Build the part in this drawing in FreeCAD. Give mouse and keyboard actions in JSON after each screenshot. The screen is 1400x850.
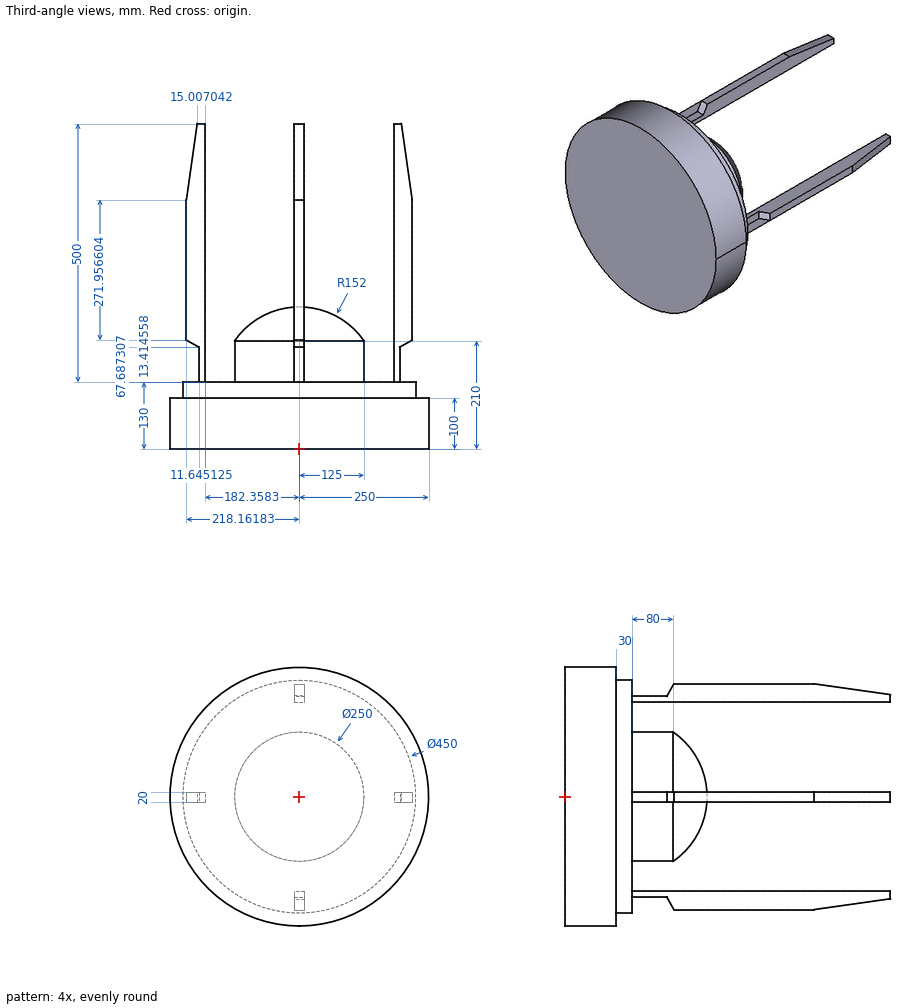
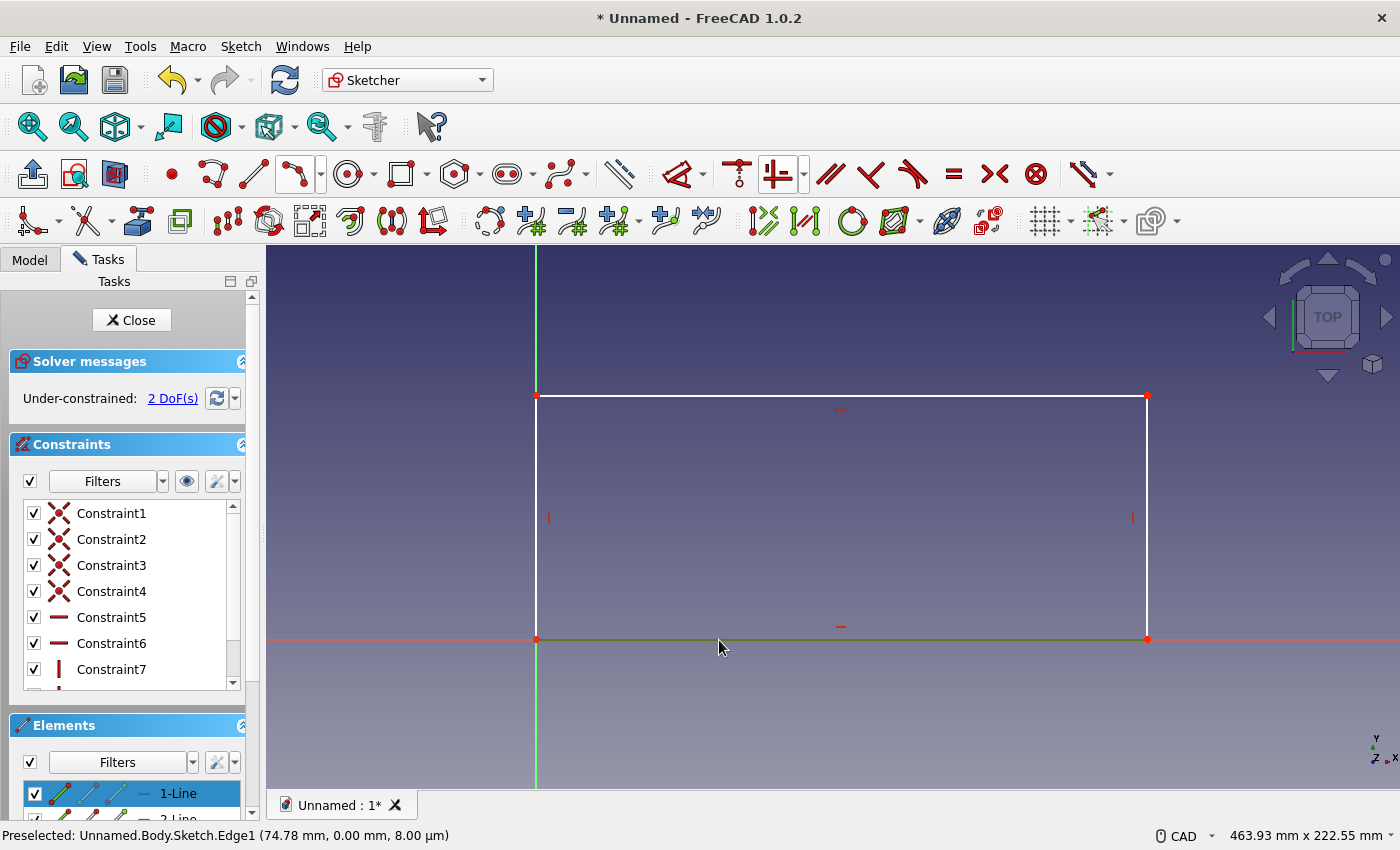
{"action": "left_click", "coordinate": [702, 174]}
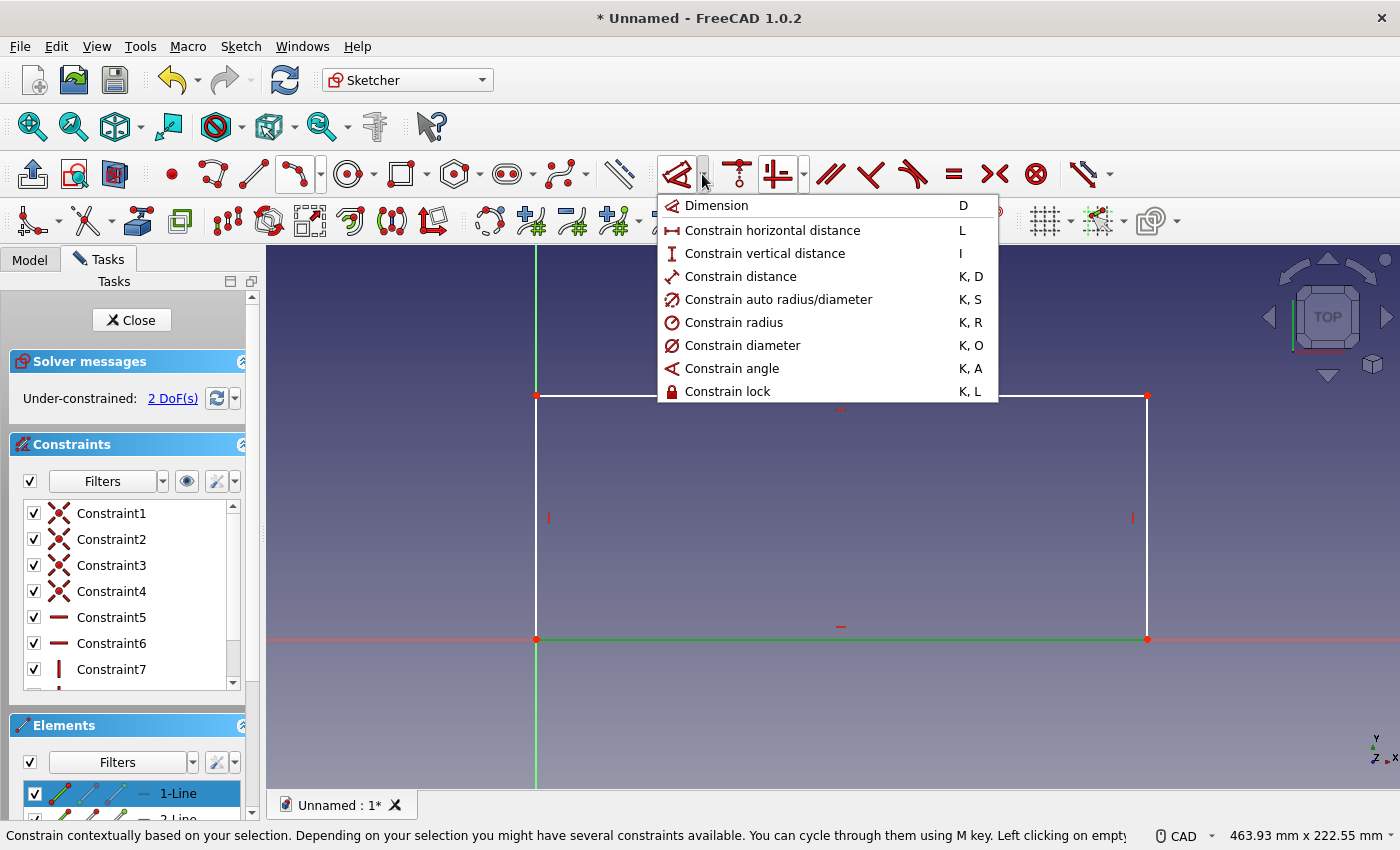
{"action": "left_click", "coordinate": [828, 230]}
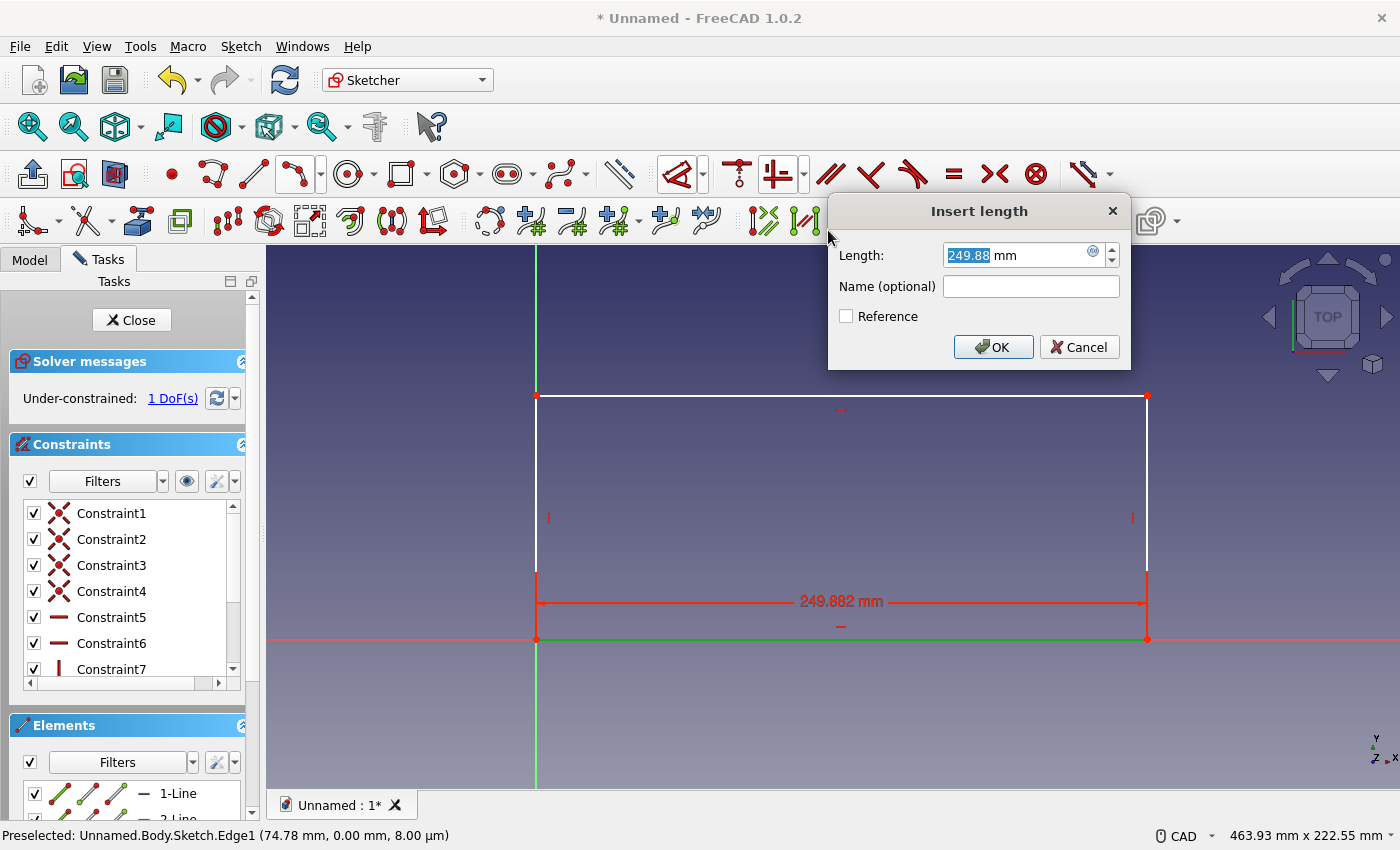
{"action": "type", "text": "250"}
{"action": "key", "text": "Return"}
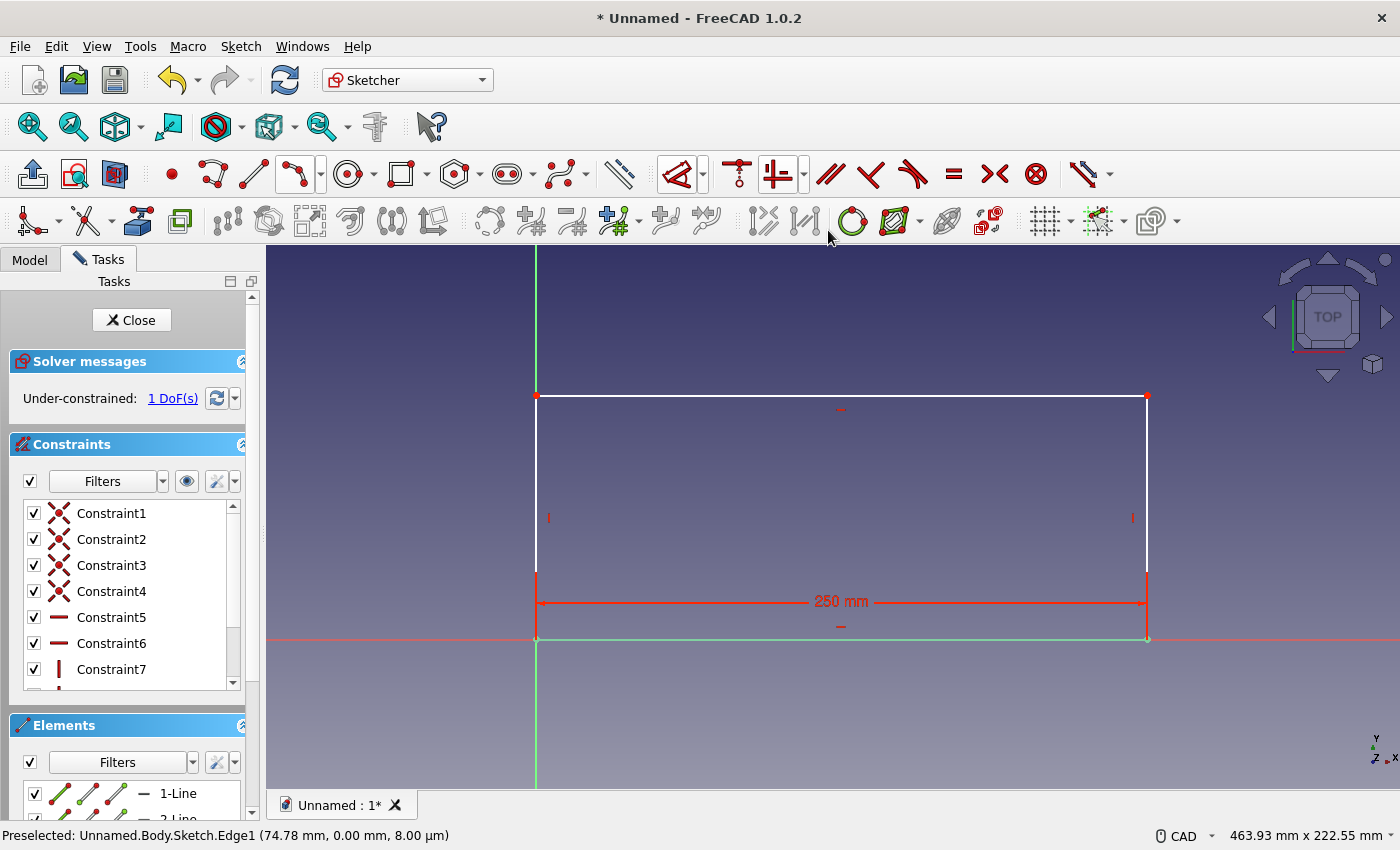
{"action": "left_click", "coordinate": [1147, 567]}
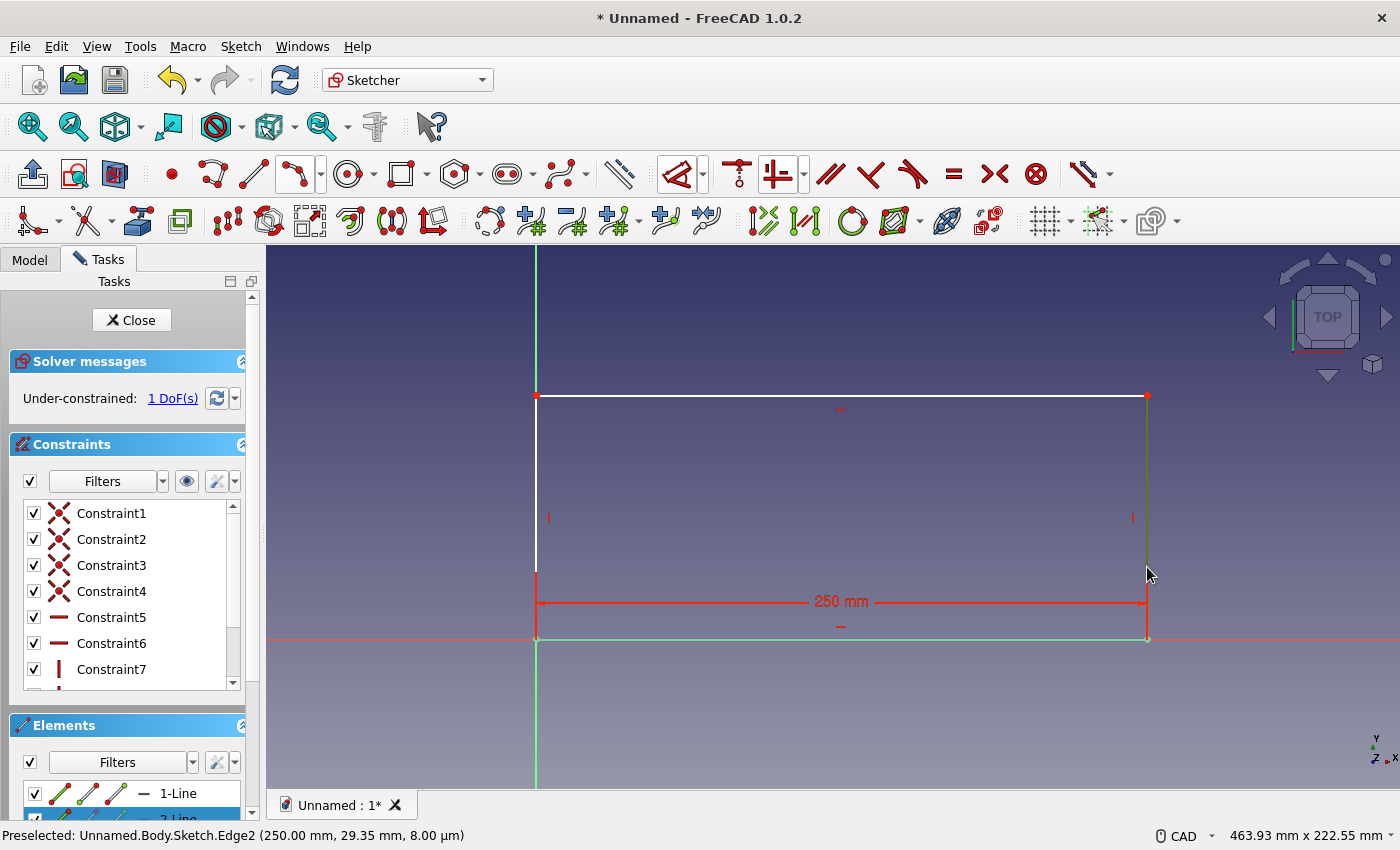
{"action": "left_click", "coordinate": [702, 174]}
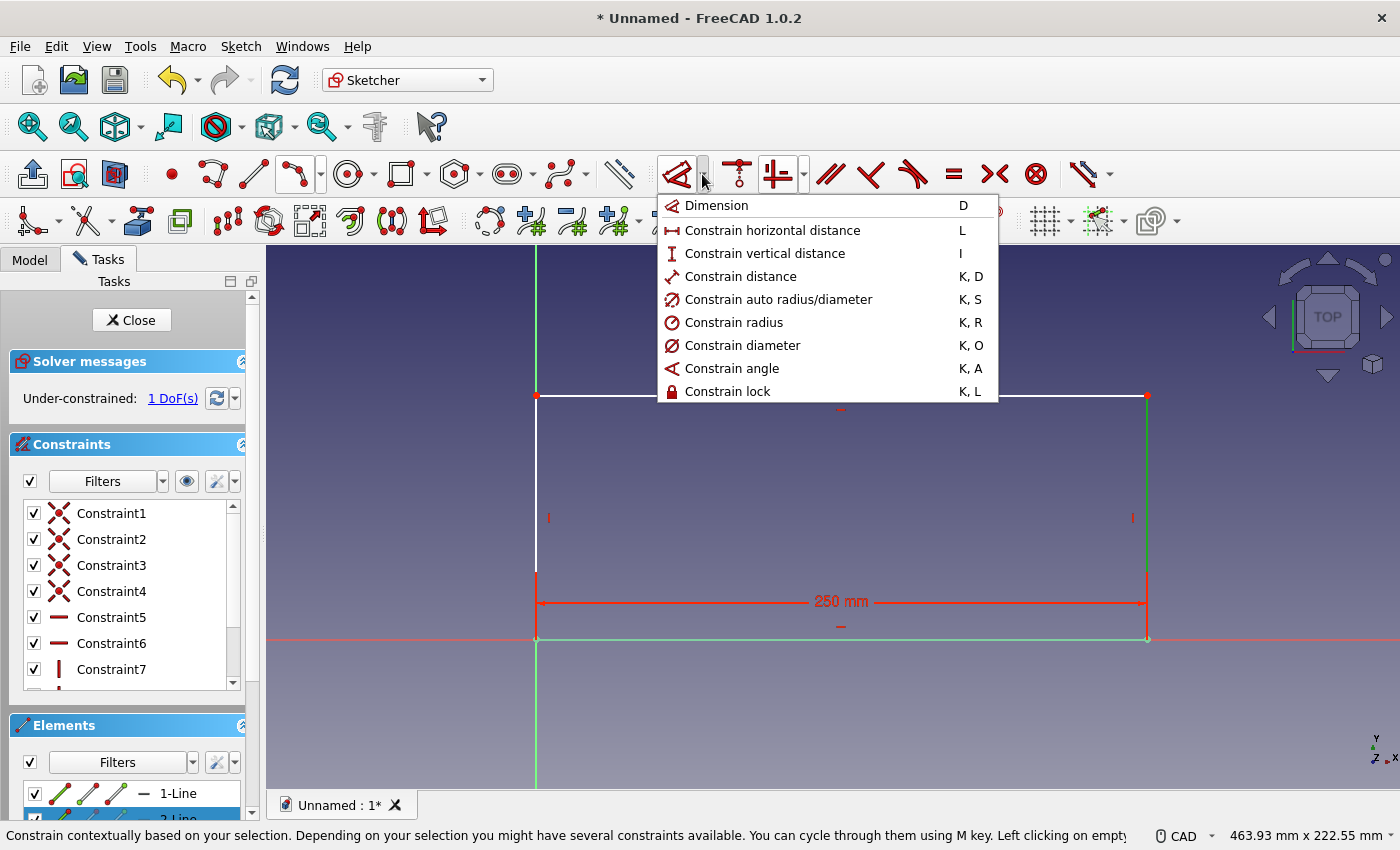
{"action": "left_click", "coordinate": [828, 254]}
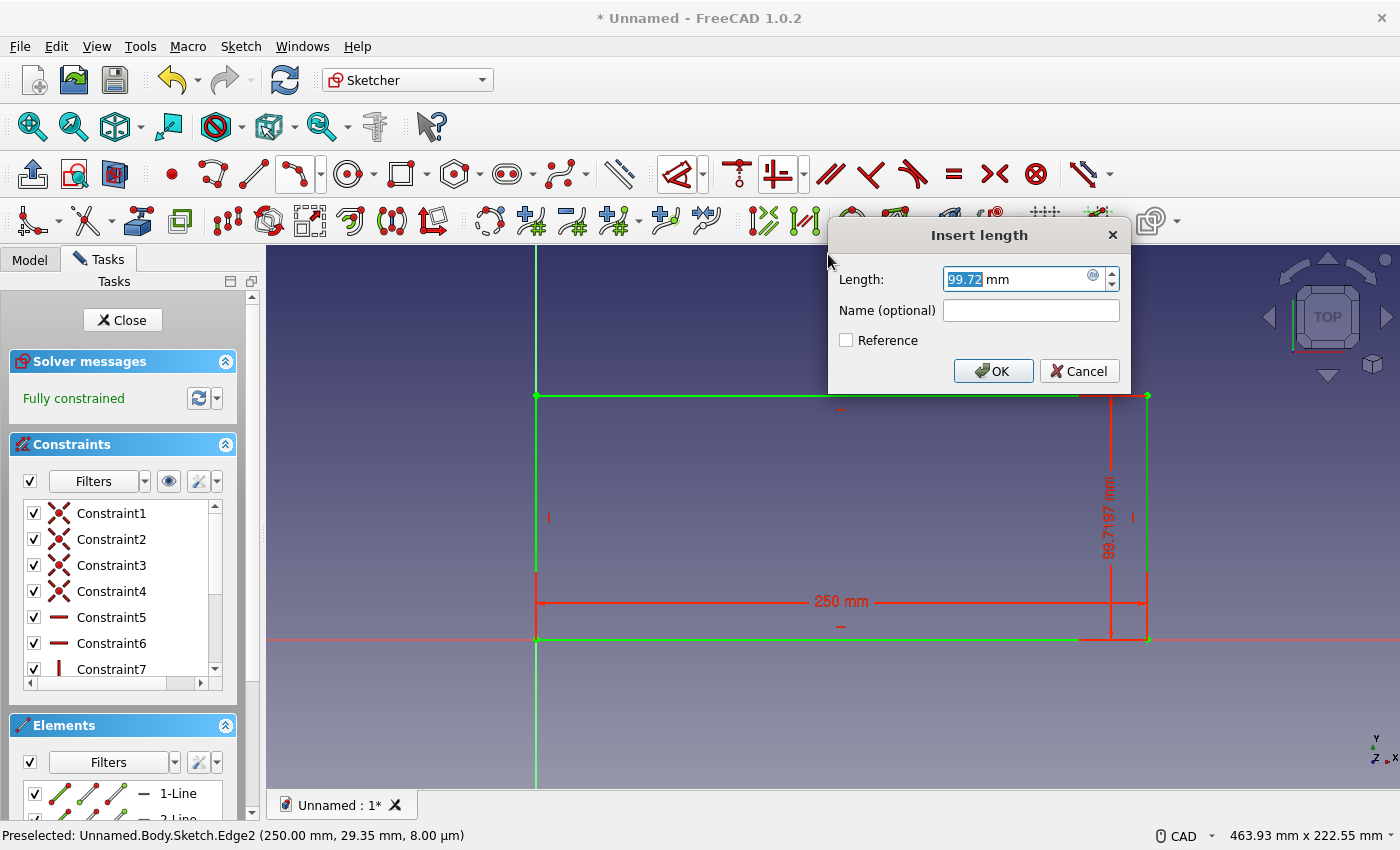
{"action": "type", "text": "100"}
{"action": "key", "text": "Return"}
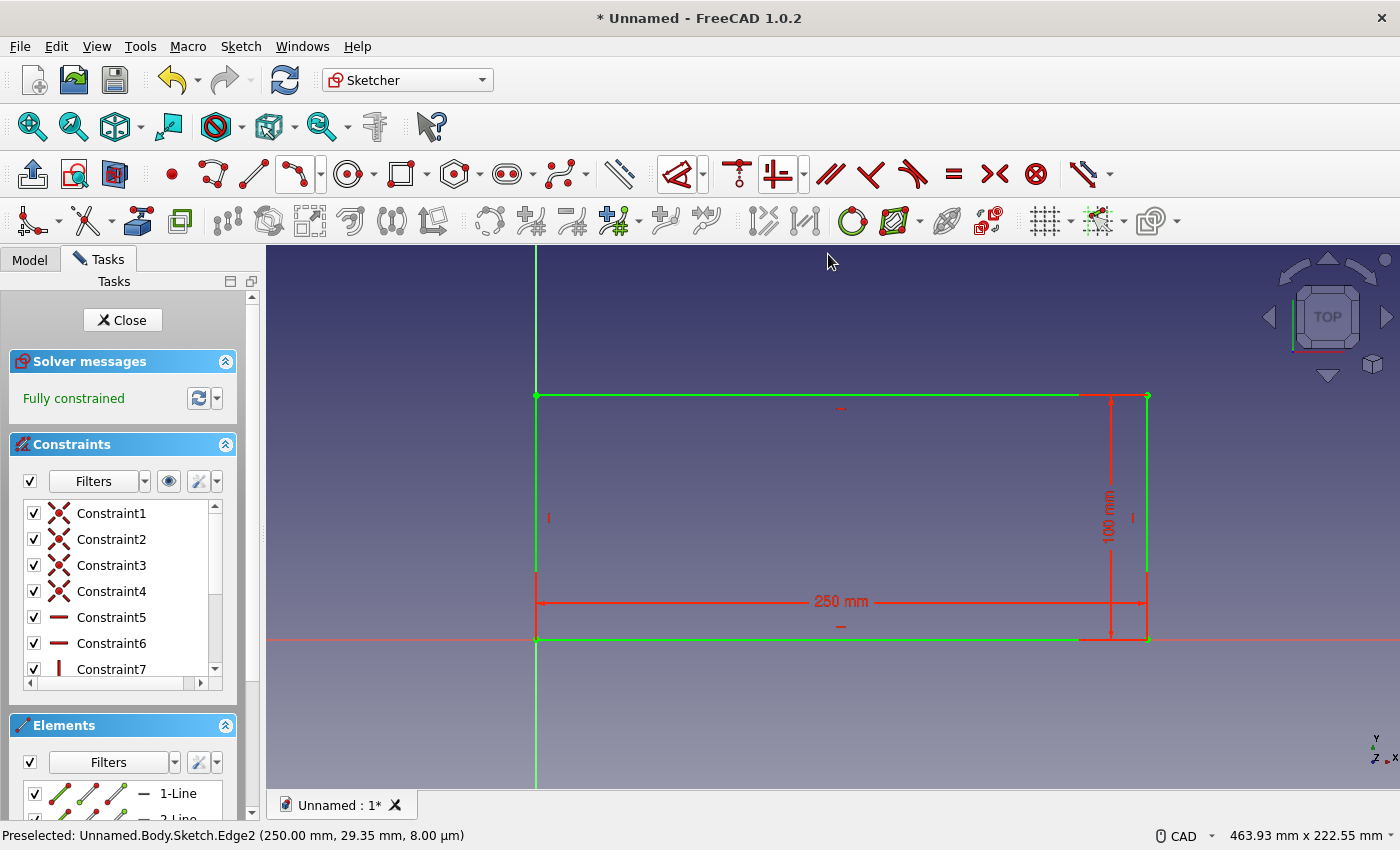
{"action": "left_click", "coordinate": [123, 320]}